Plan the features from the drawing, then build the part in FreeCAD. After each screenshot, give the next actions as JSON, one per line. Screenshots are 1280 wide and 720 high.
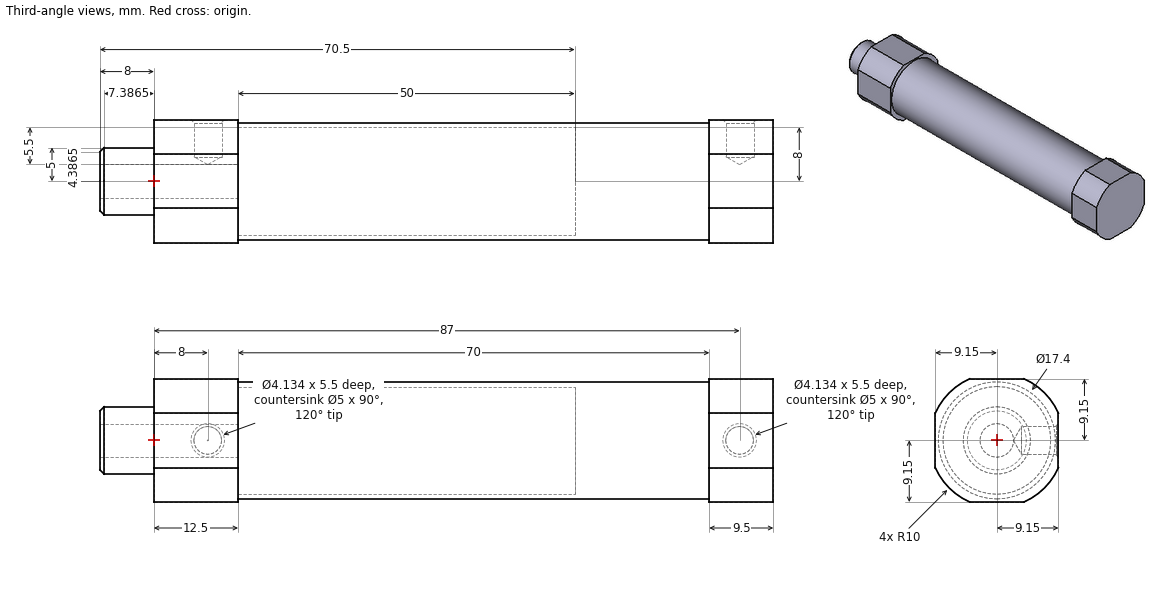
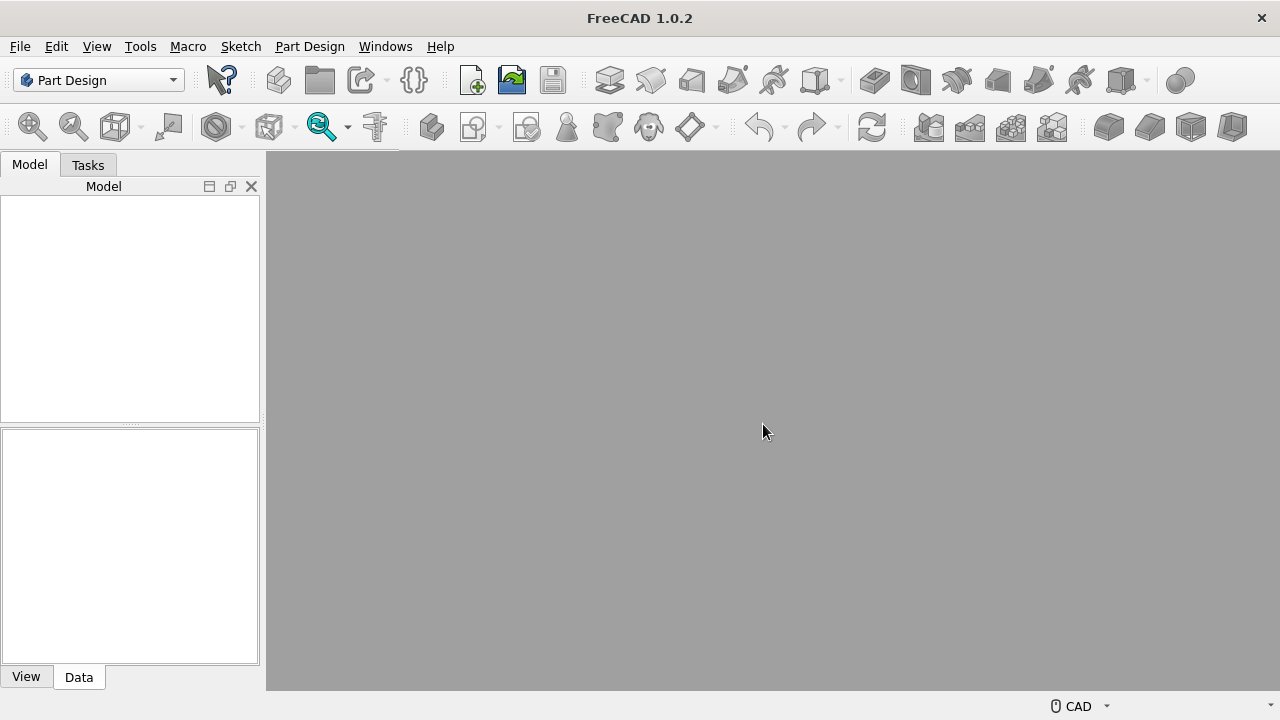
{"action": "left_click", "coordinate": [471, 80]}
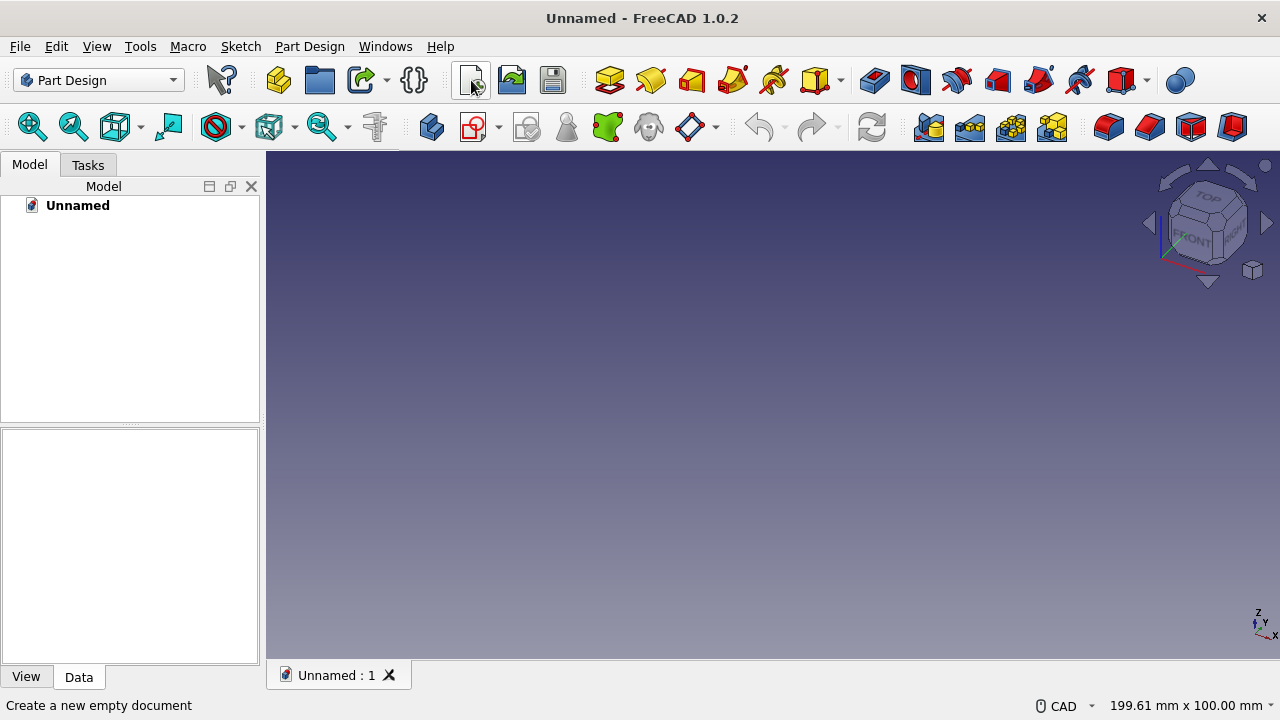
{"action": "left_click", "coordinate": [472, 128]}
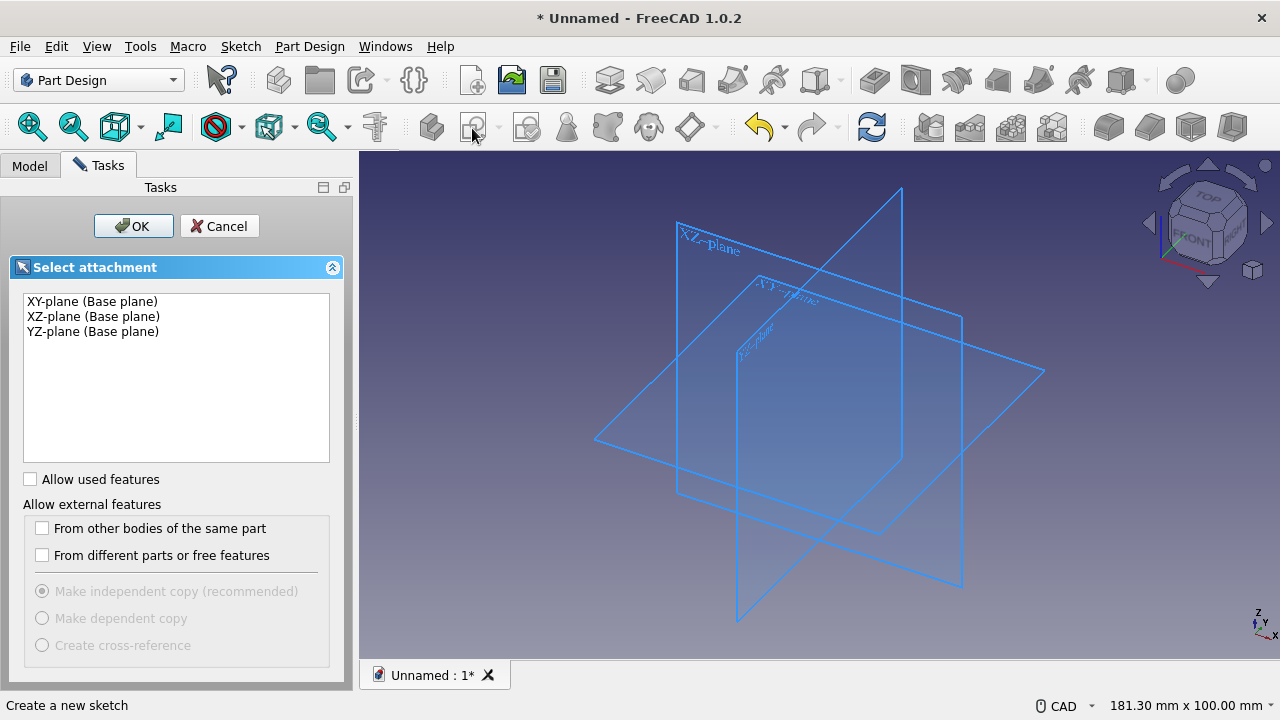
{"action": "left_click", "coordinate": [84, 302]}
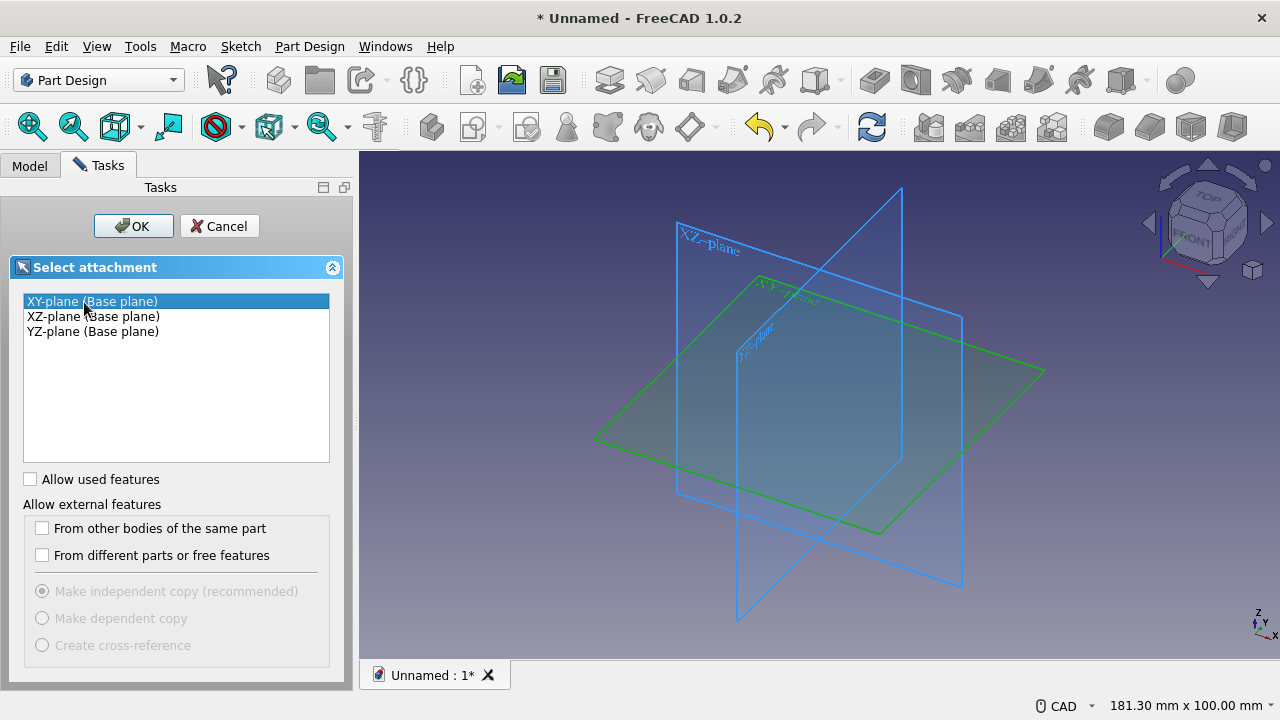
{"action": "left_click", "coordinate": [134, 226]}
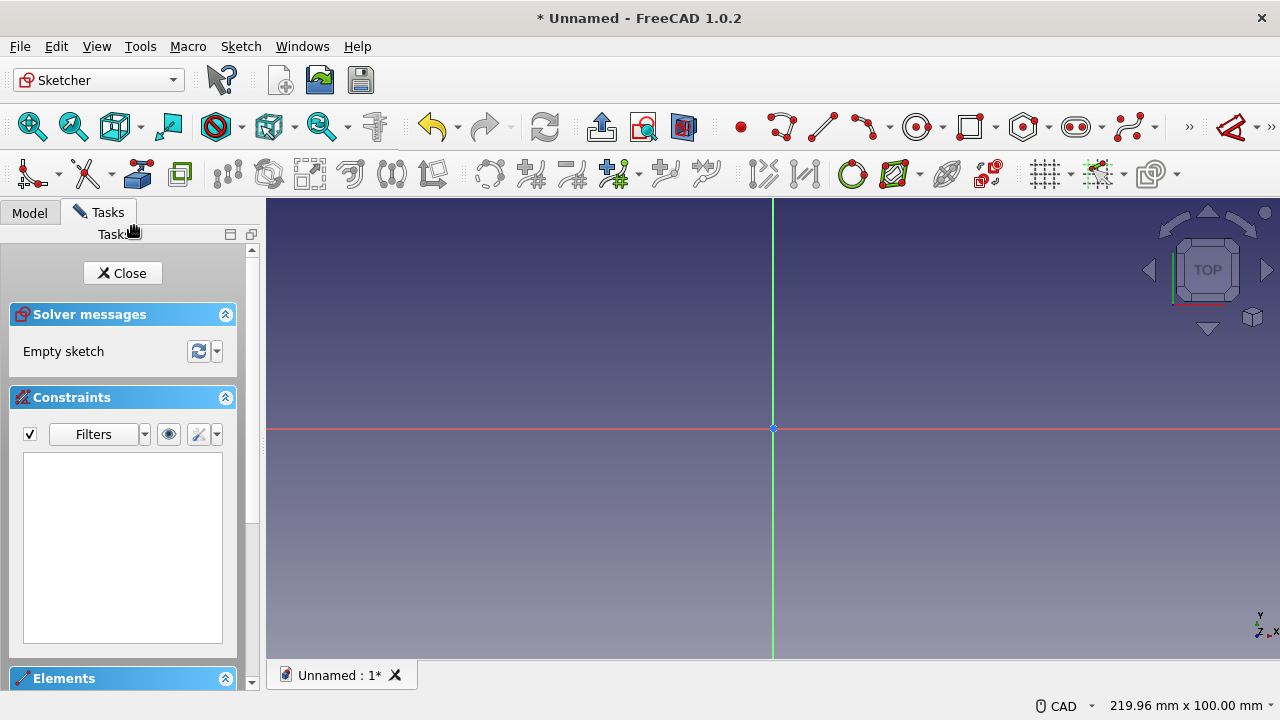
{"action": "scroll", "coordinate": [759, 416], "scroll_direction": "up", "scroll_amount": 13}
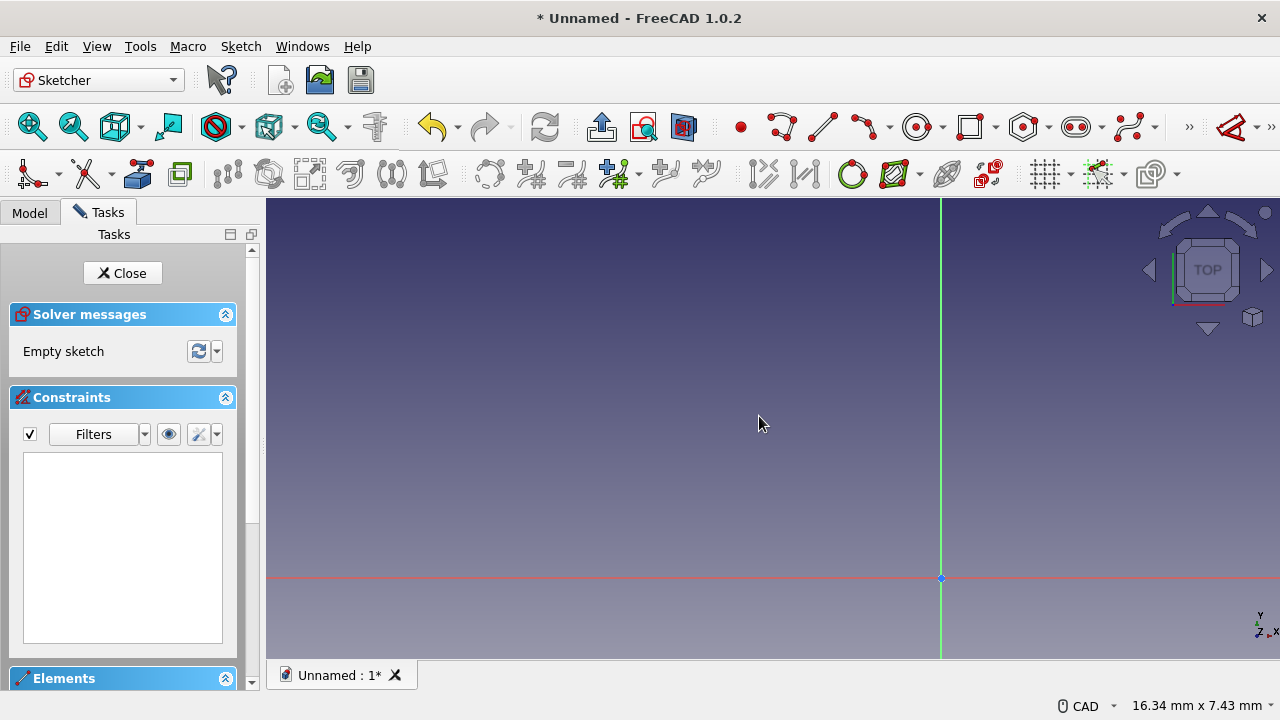
{"action": "left_click", "coordinate": [782, 128]}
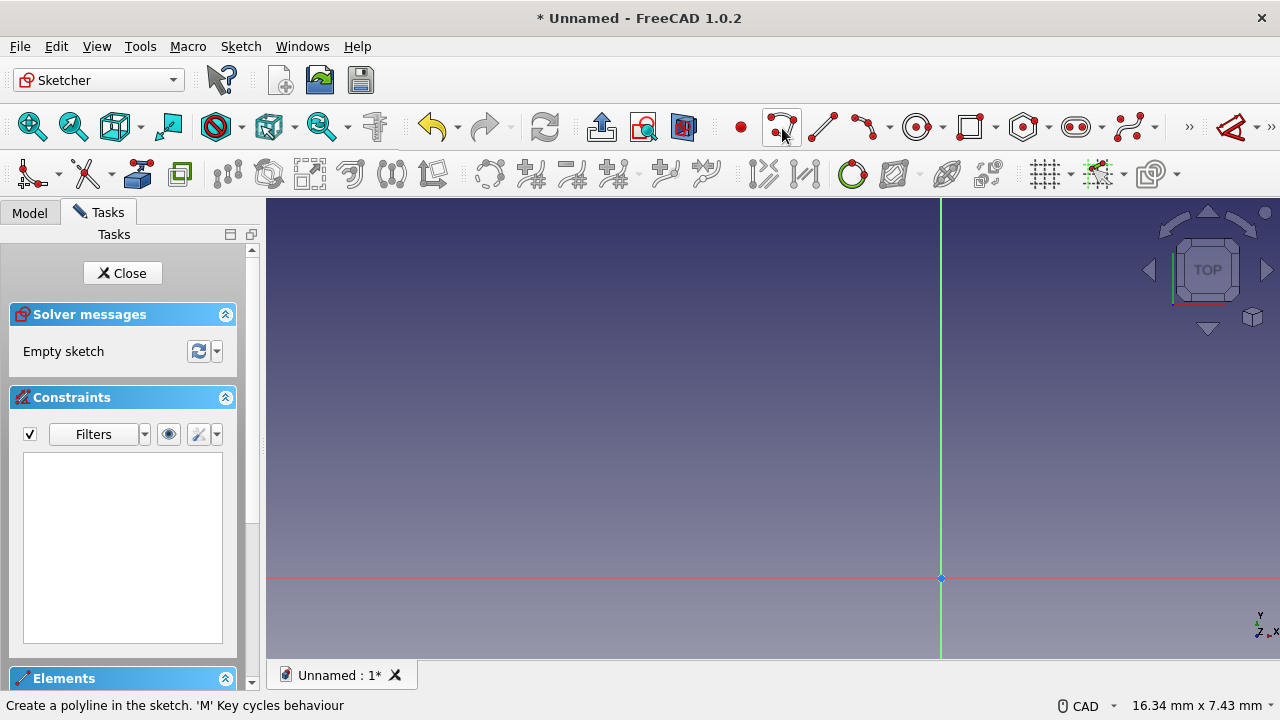
{"action": "left_click", "coordinate": [941, 578]}
{"action": "left_click", "coordinate": [932, 268]}
{"action": "left_click", "coordinate": [483, 268]}
{"action": "left_click", "coordinate": [445, 306]}
{"action": "left_click", "coordinate": [445, 569]}
{"action": "left_click", "coordinate": [941, 578]}
{"action": "key", "text": "Escape"}
{"action": "key", "text": "Escape"}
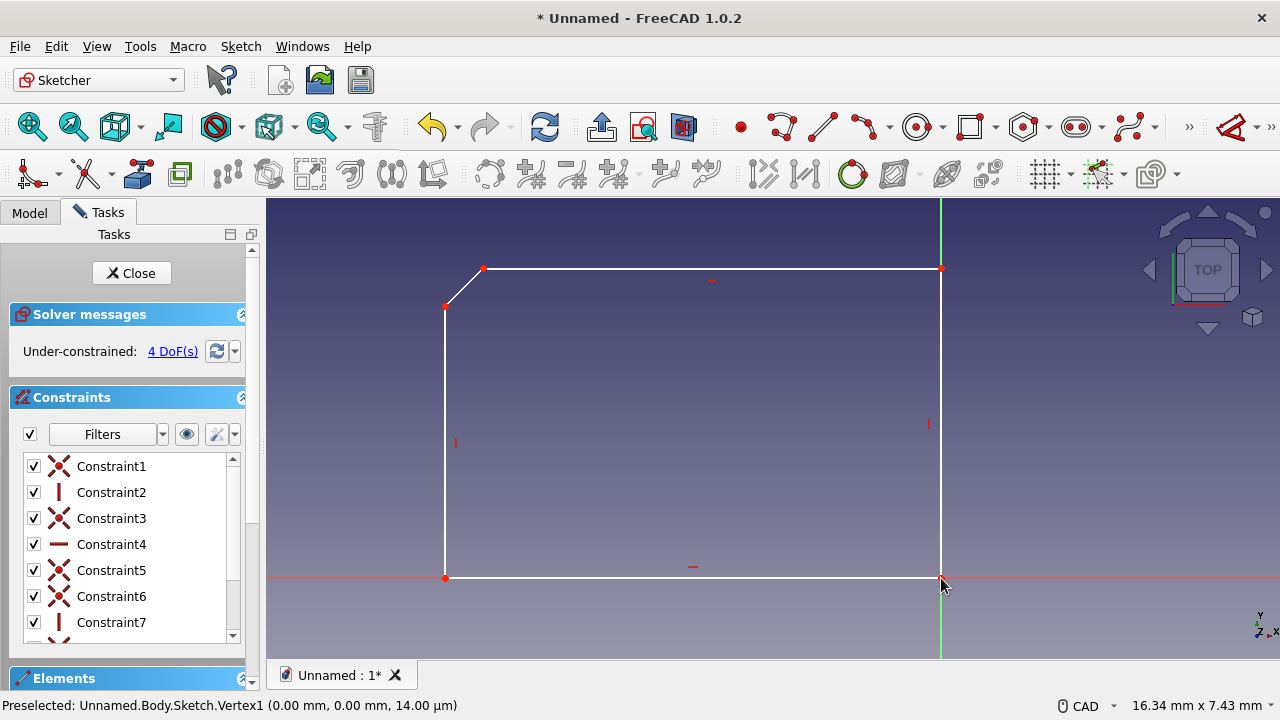
{"action": "key", "text": "d"}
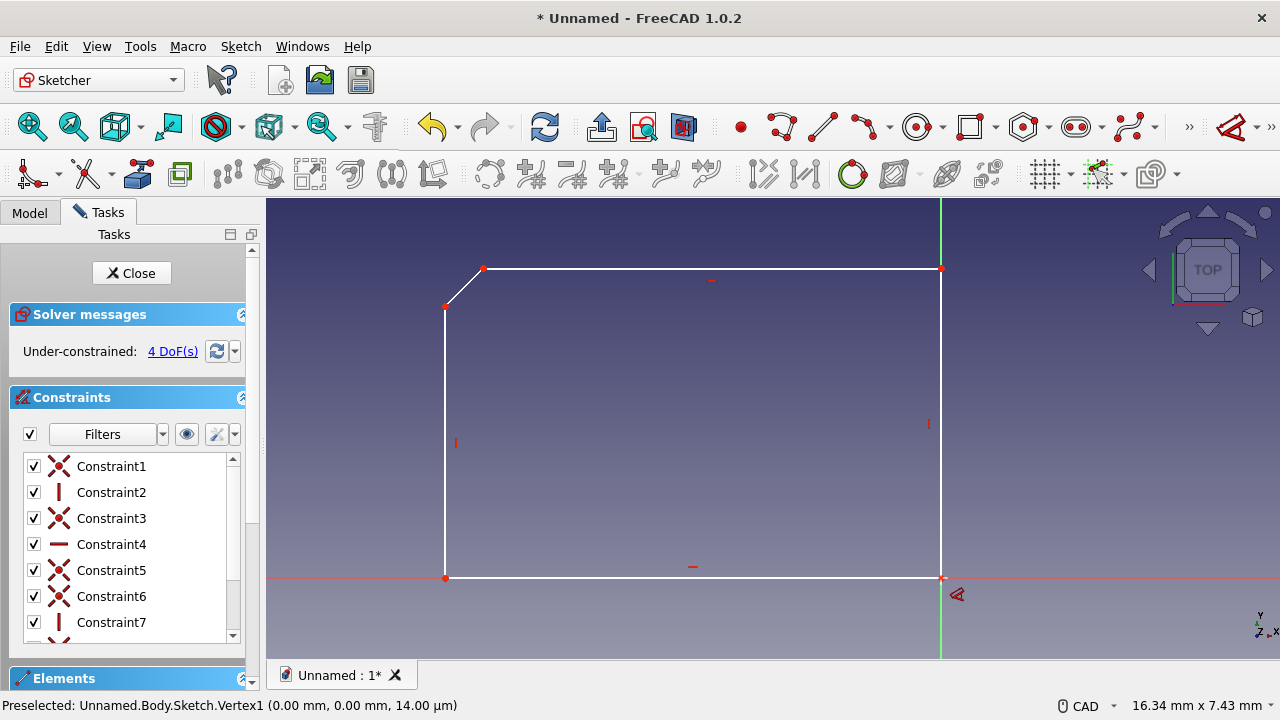
{"action": "left_click", "coordinate": [941, 486]}
{"action": "left_click", "coordinate": [975, 424]}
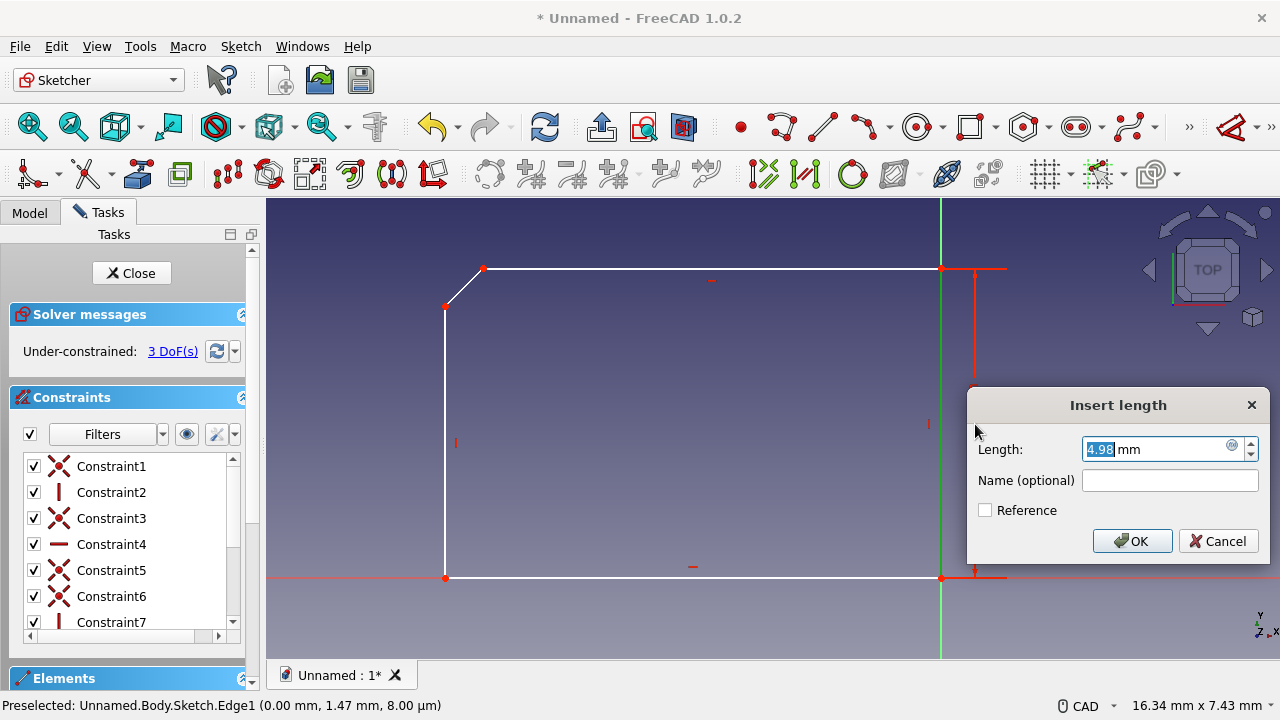
{"action": "type", "text": "5"}
{"action": "key", "text": "Return"}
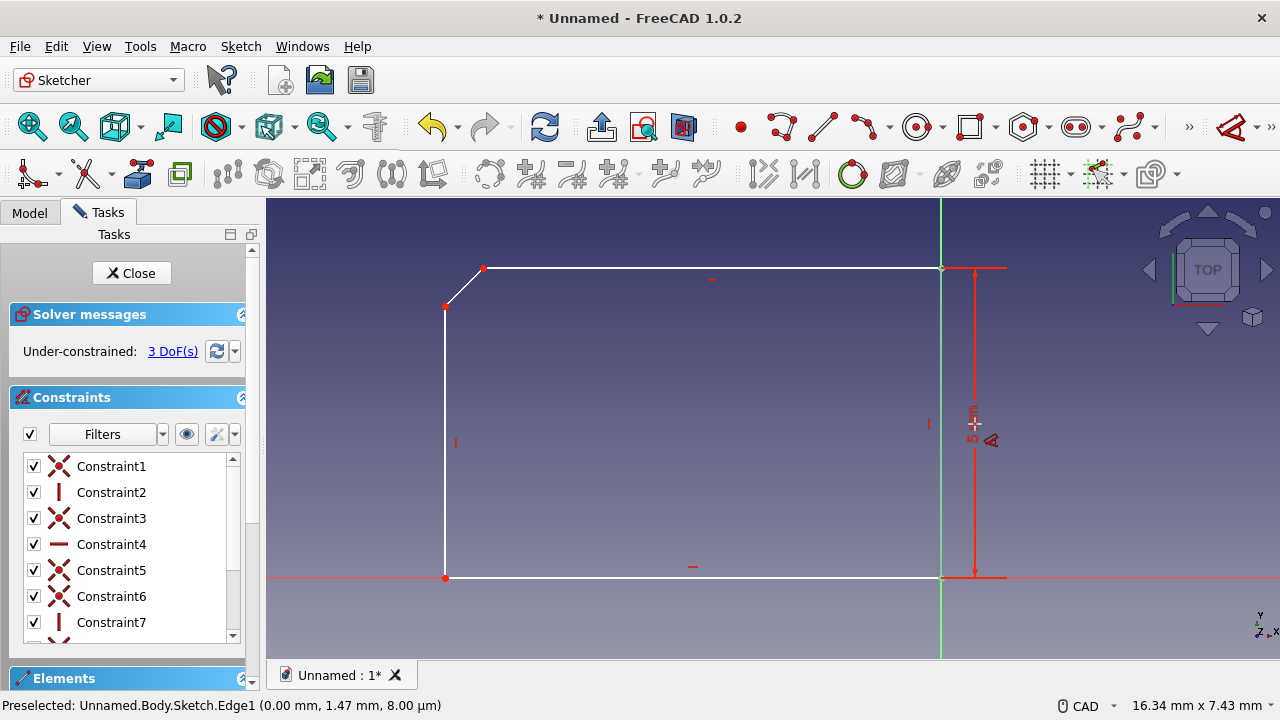
{"action": "left_click", "coordinate": [594, 578]}
{"action": "left_click", "coordinate": [693, 612]}